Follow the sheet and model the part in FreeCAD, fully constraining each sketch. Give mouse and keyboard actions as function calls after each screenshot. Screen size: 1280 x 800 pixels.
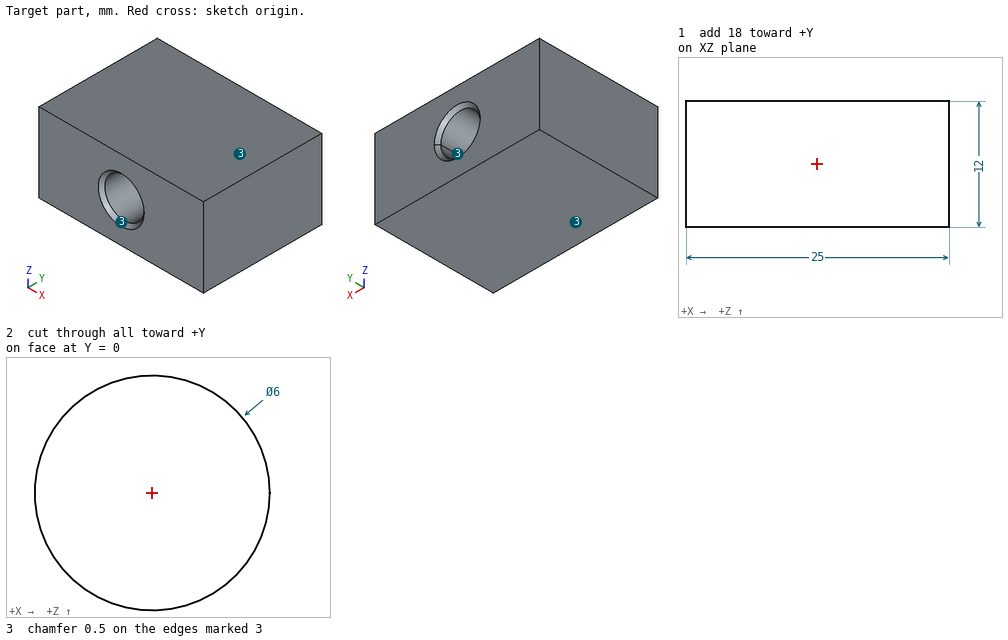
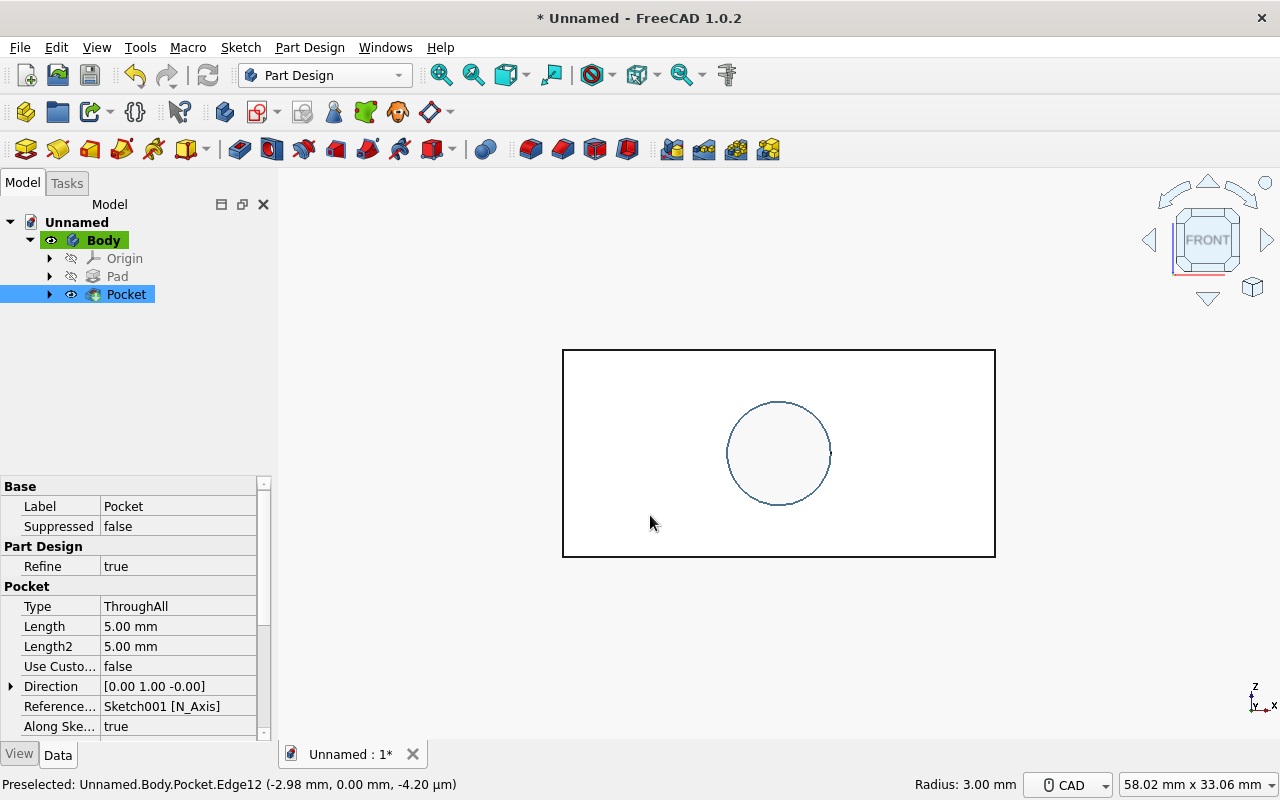
key(v)
key(f)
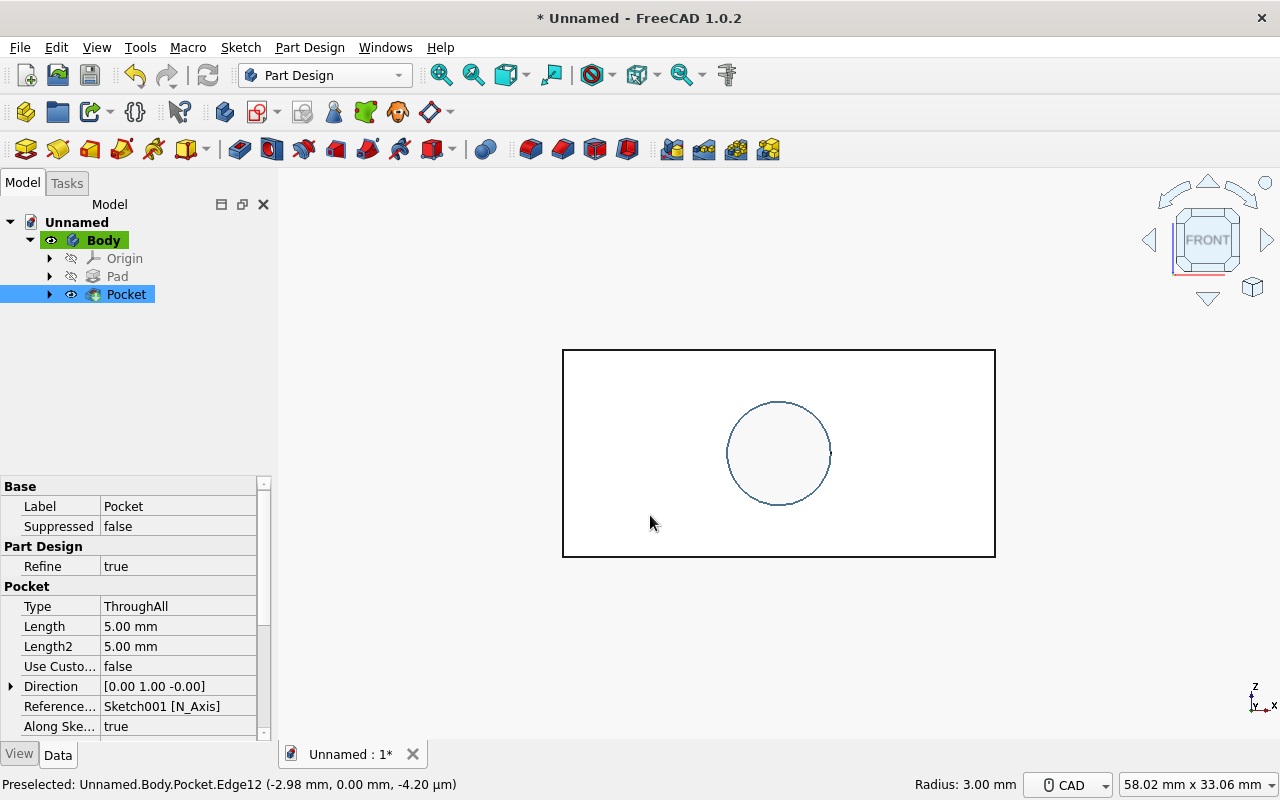
key(3)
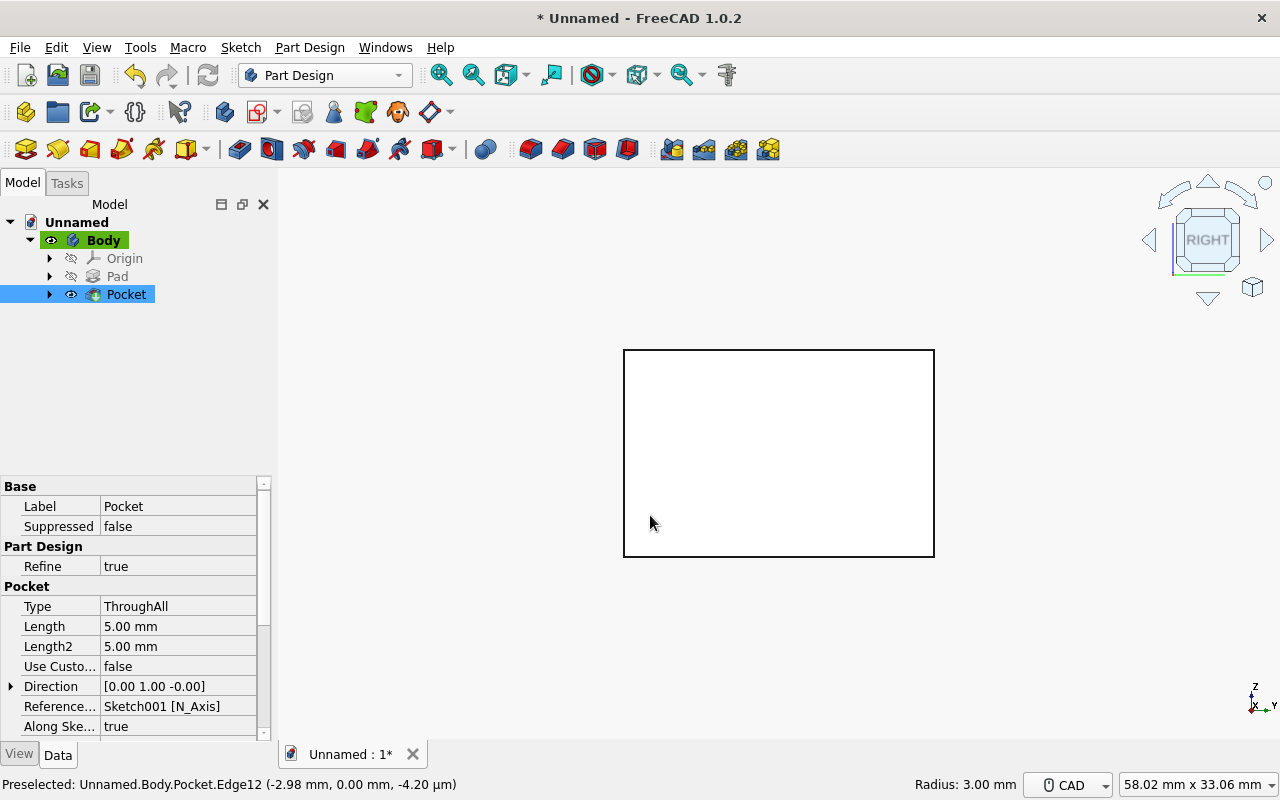
click(442, 76)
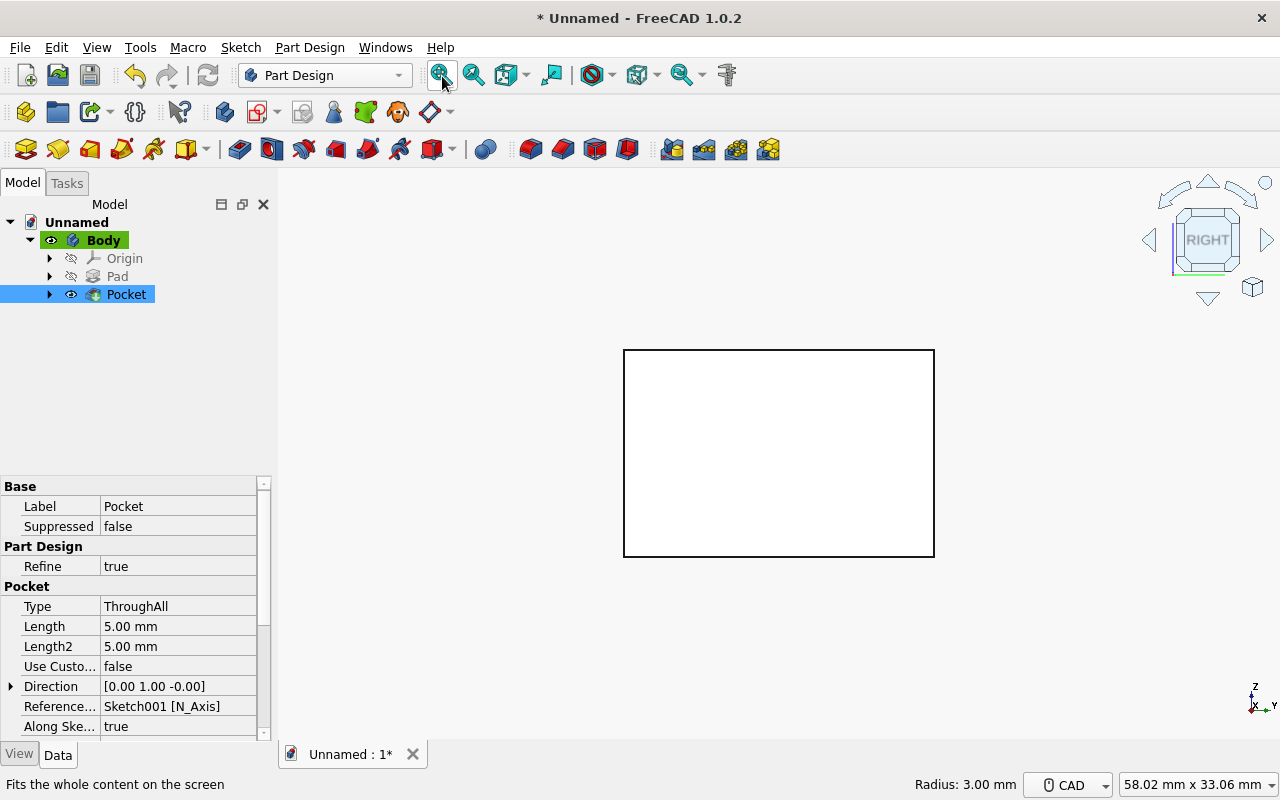
key(5)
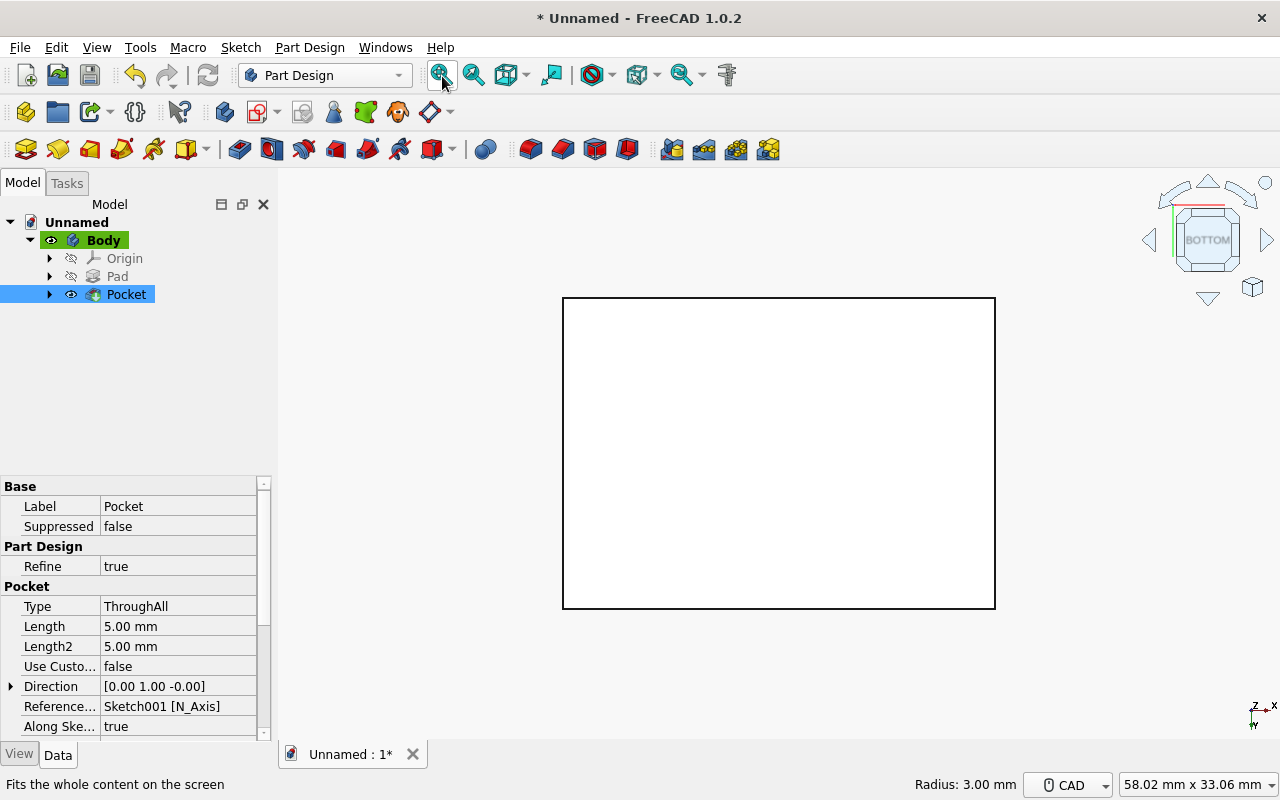
key(4)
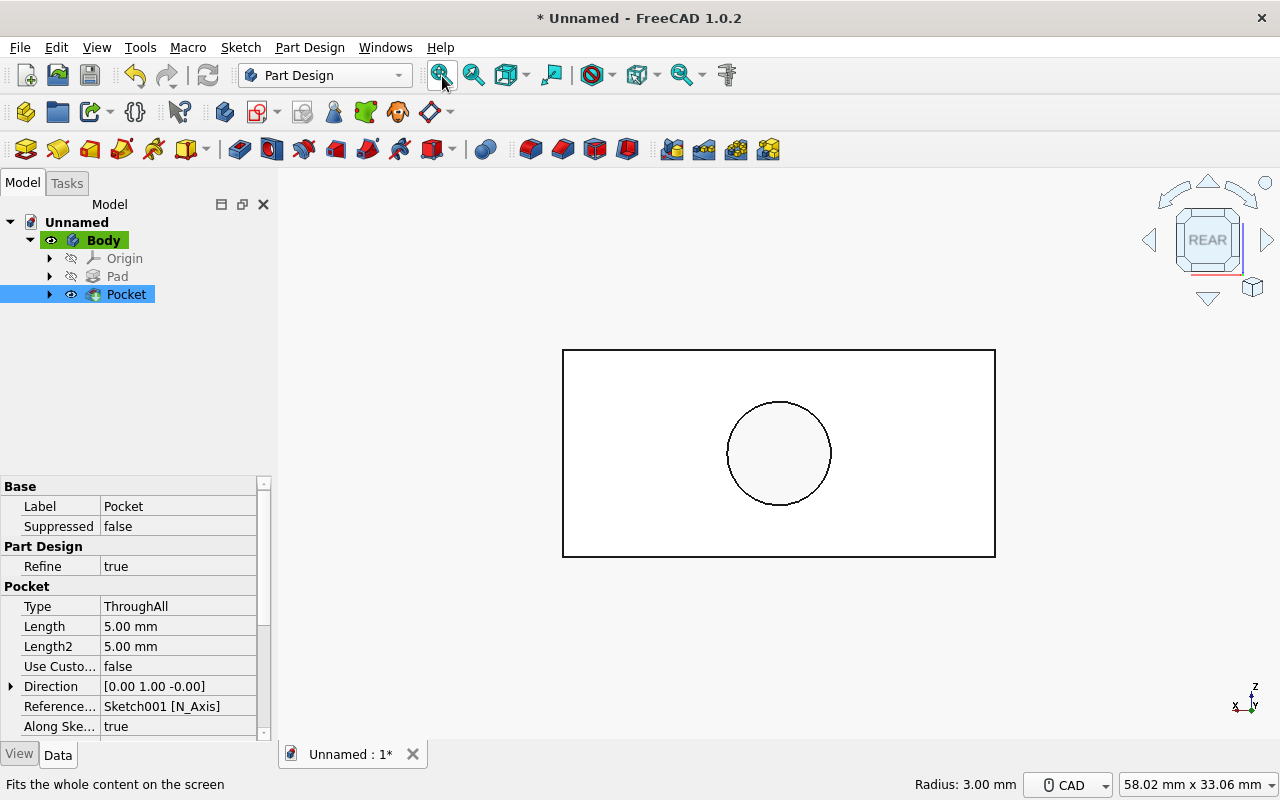
click(442, 76)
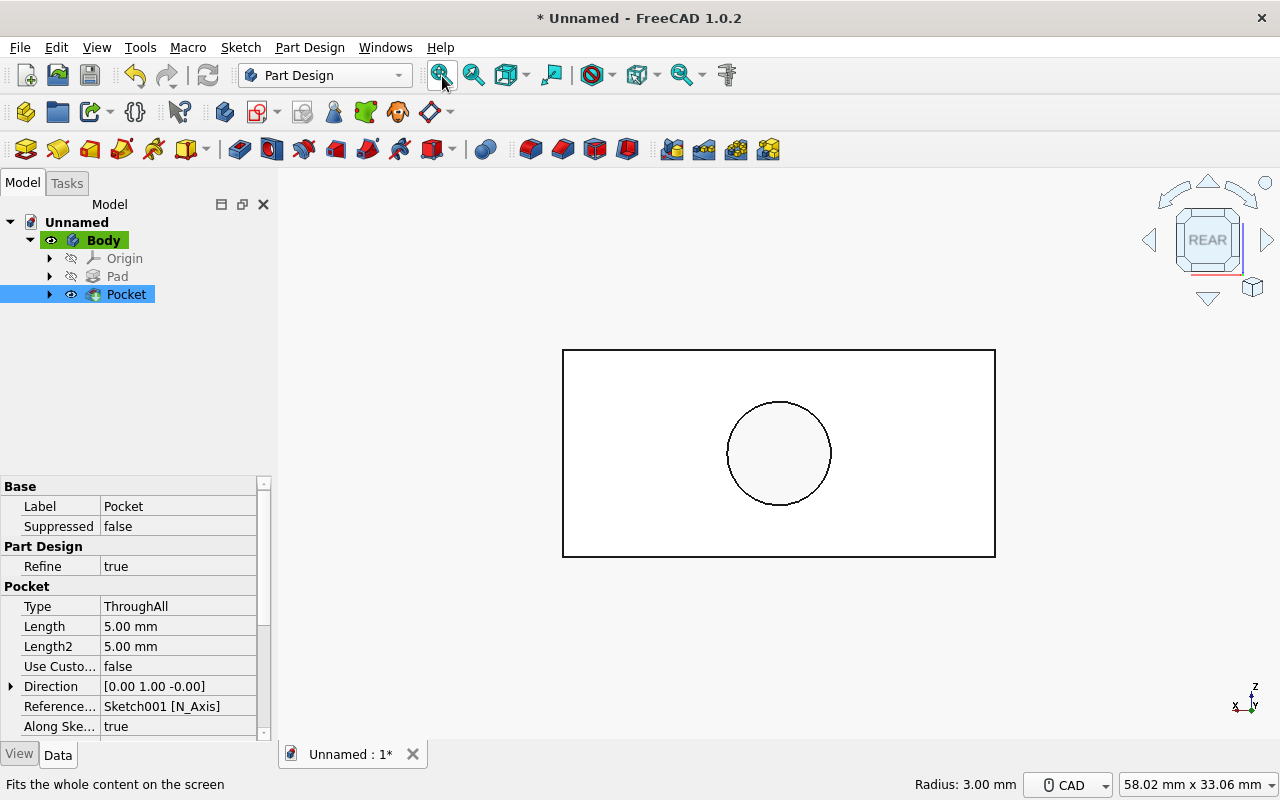
click(831, 453, ctrl)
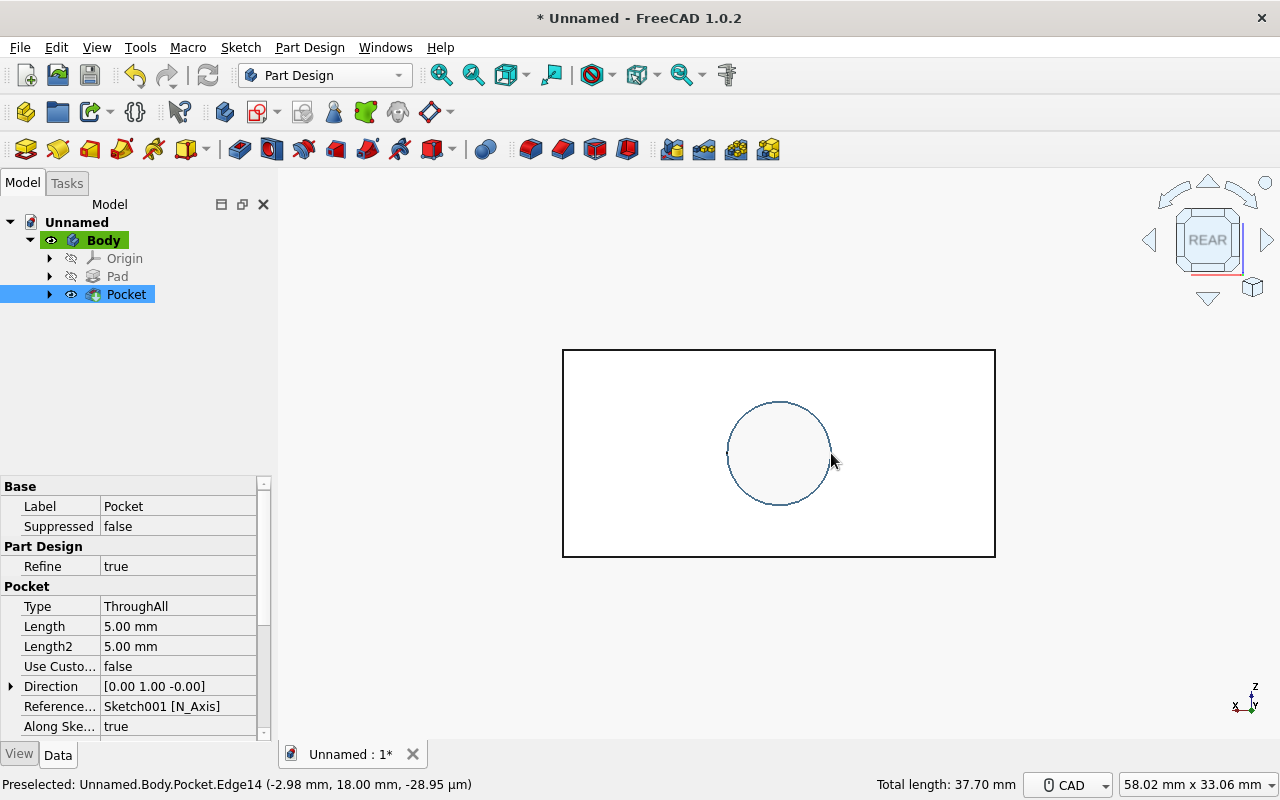
click(564, 150)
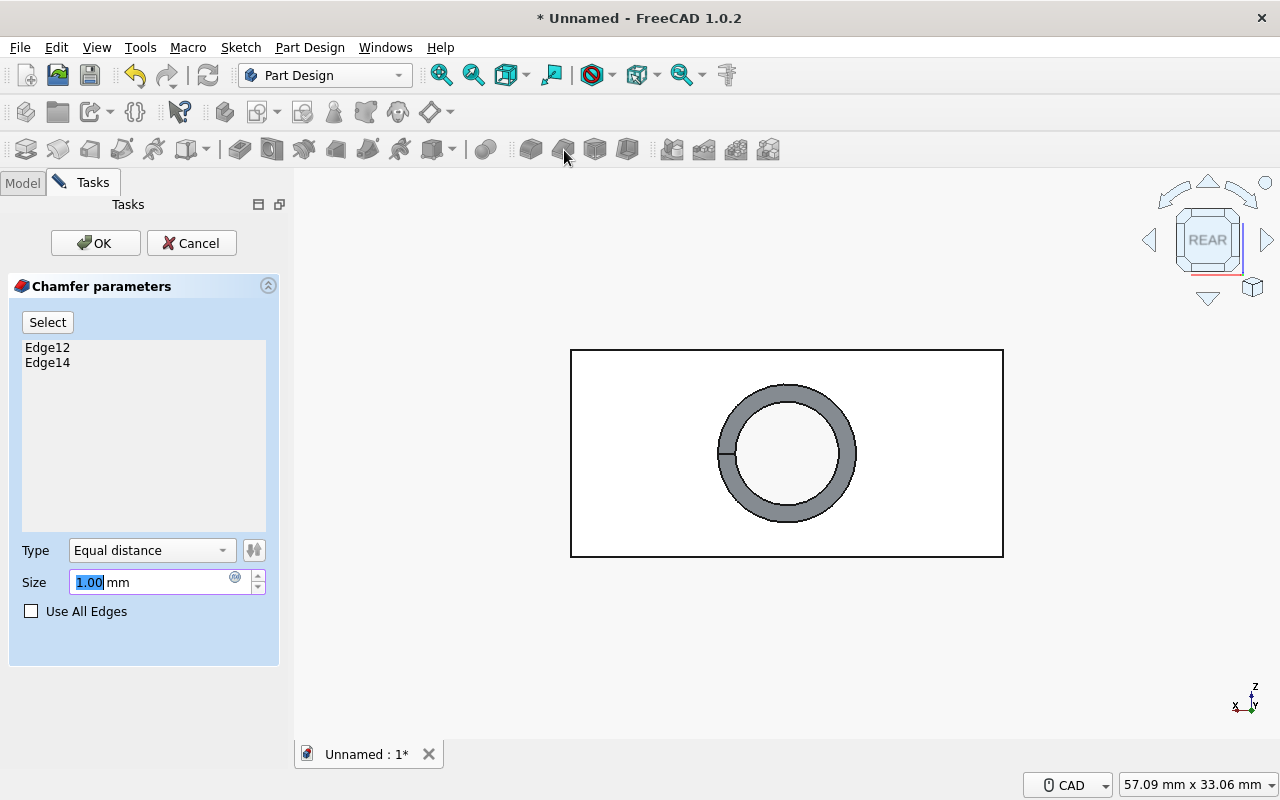
text(0.5)
key(Tab)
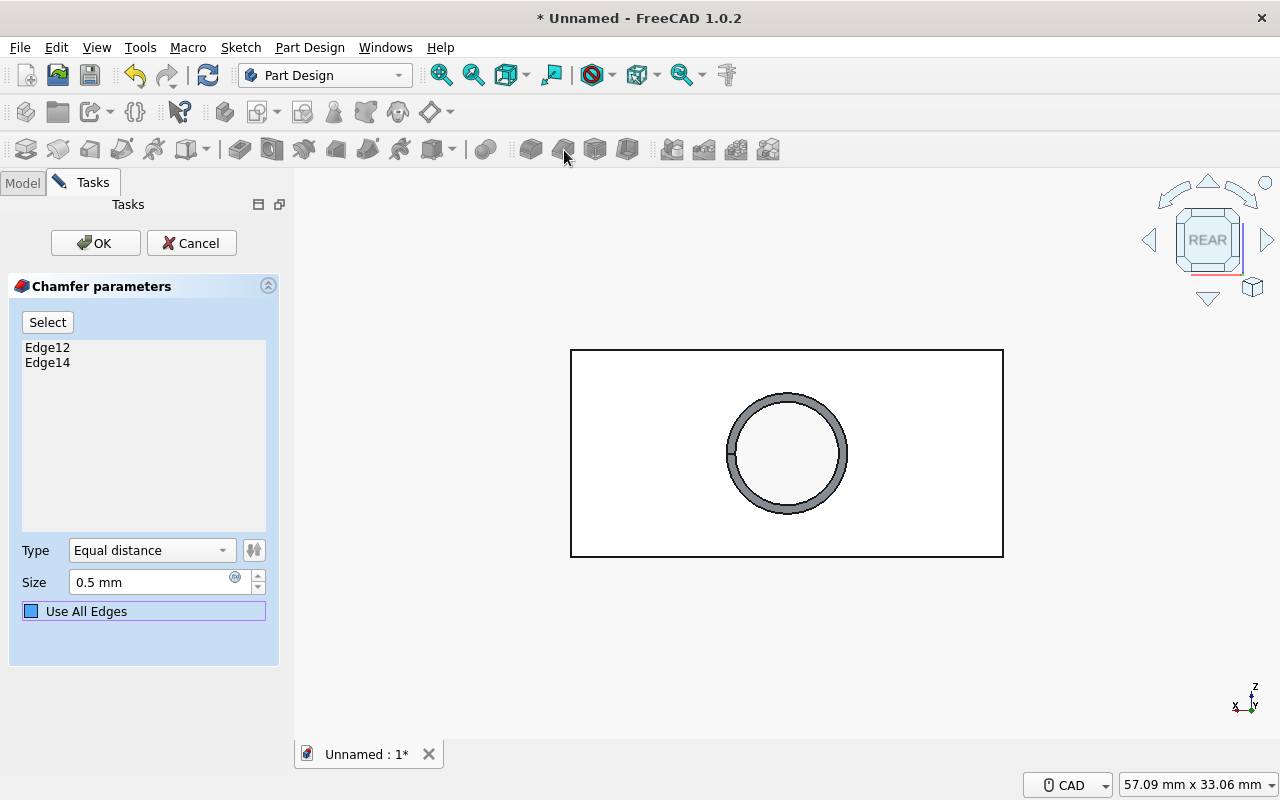
click(96, 243)